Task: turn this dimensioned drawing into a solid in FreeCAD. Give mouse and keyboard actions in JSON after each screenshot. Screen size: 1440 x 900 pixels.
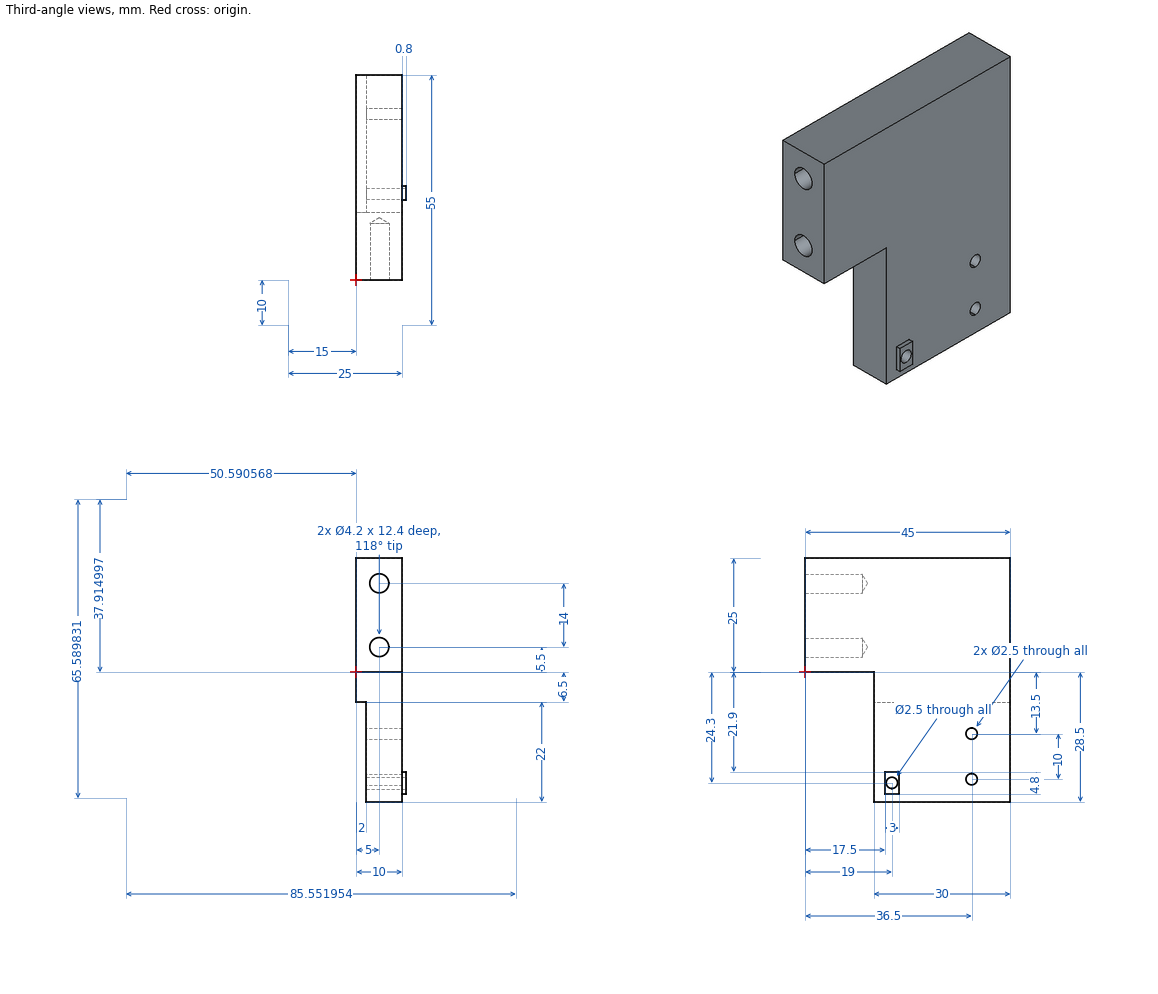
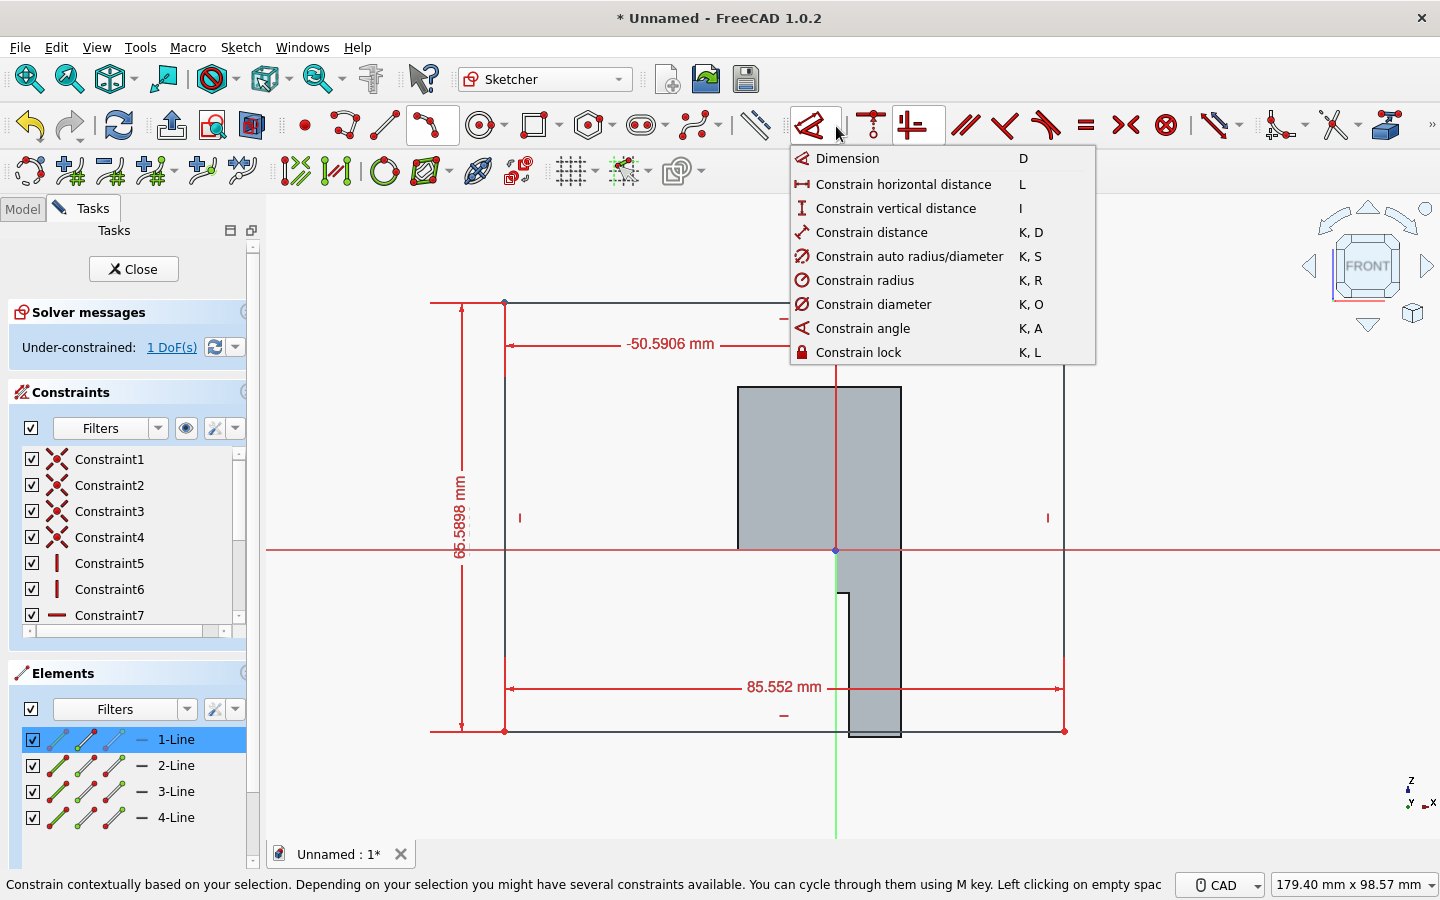
{"action": "left_click", "coordinate": [943, 208]}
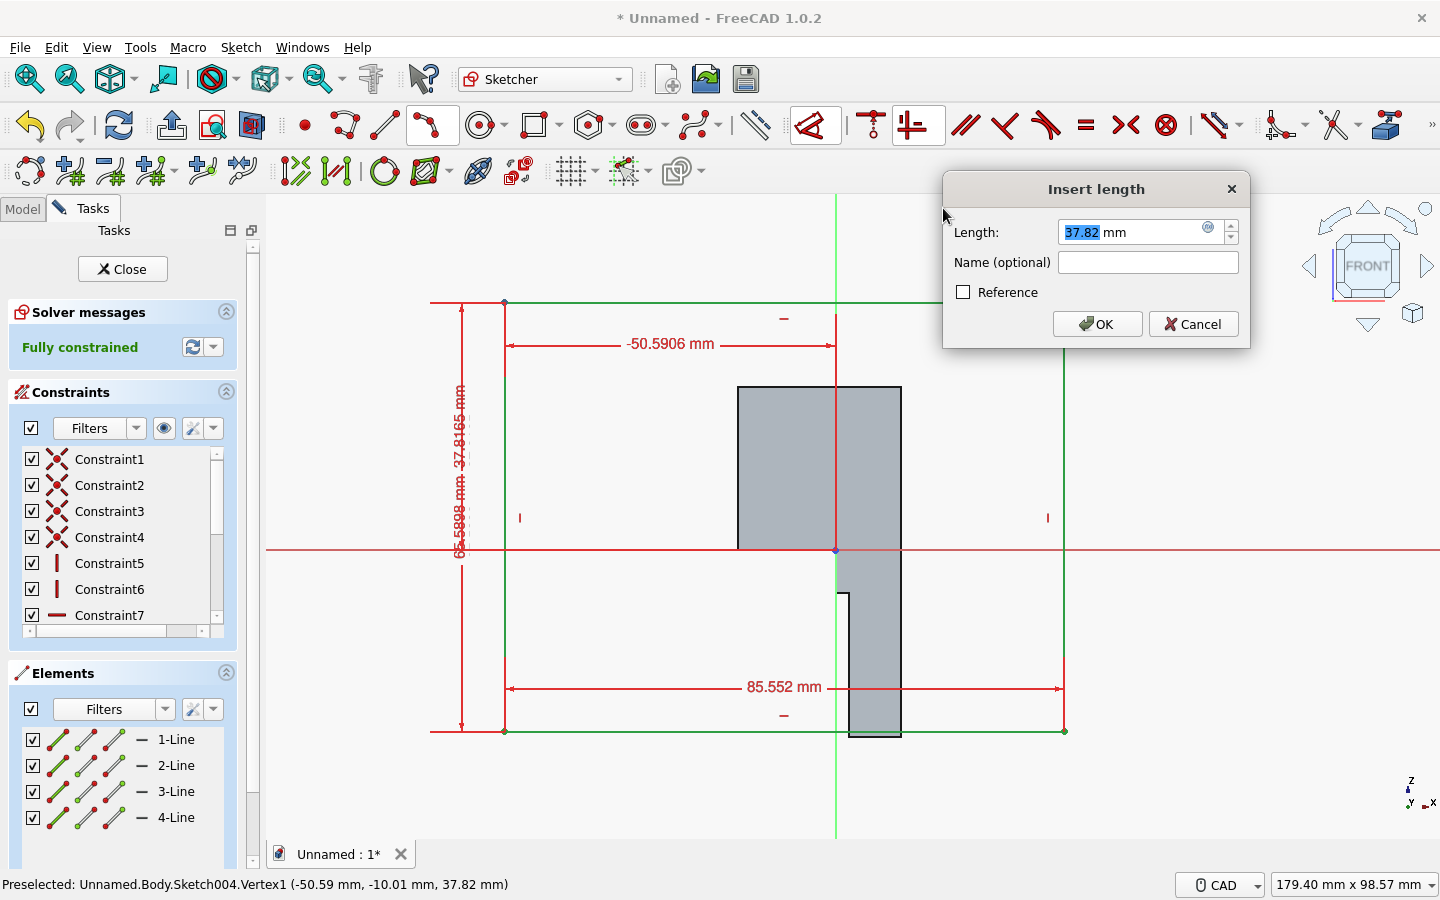
{"action": "type", "text": "37.914997"}
{"action": "key", "text": "Return"}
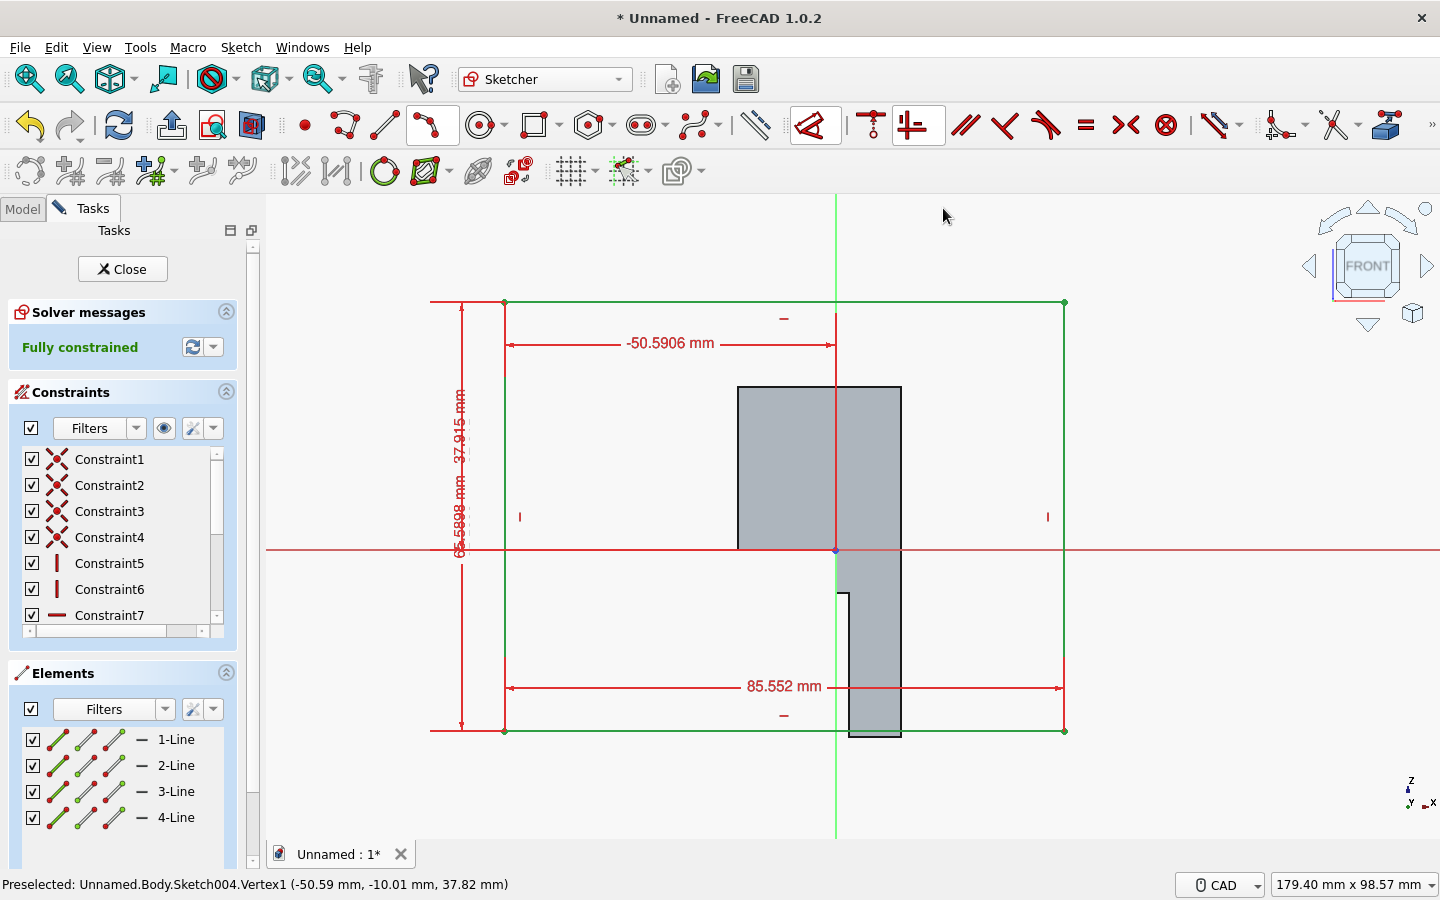
{"action": "left_click", "coordinate": [123, 269]}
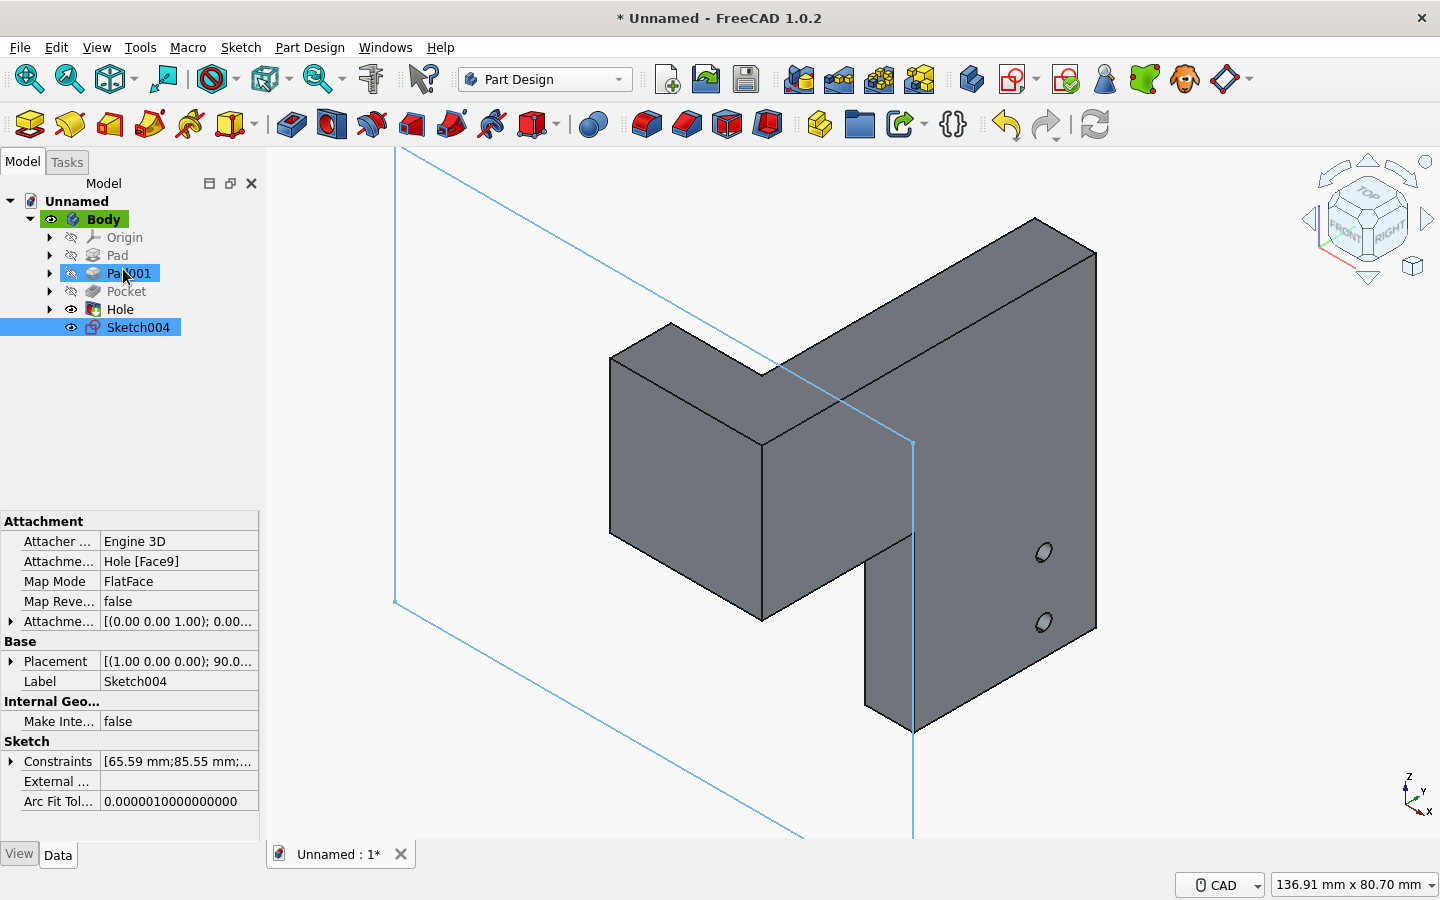
{"action": "left_click", "coordinate": [292, 124]}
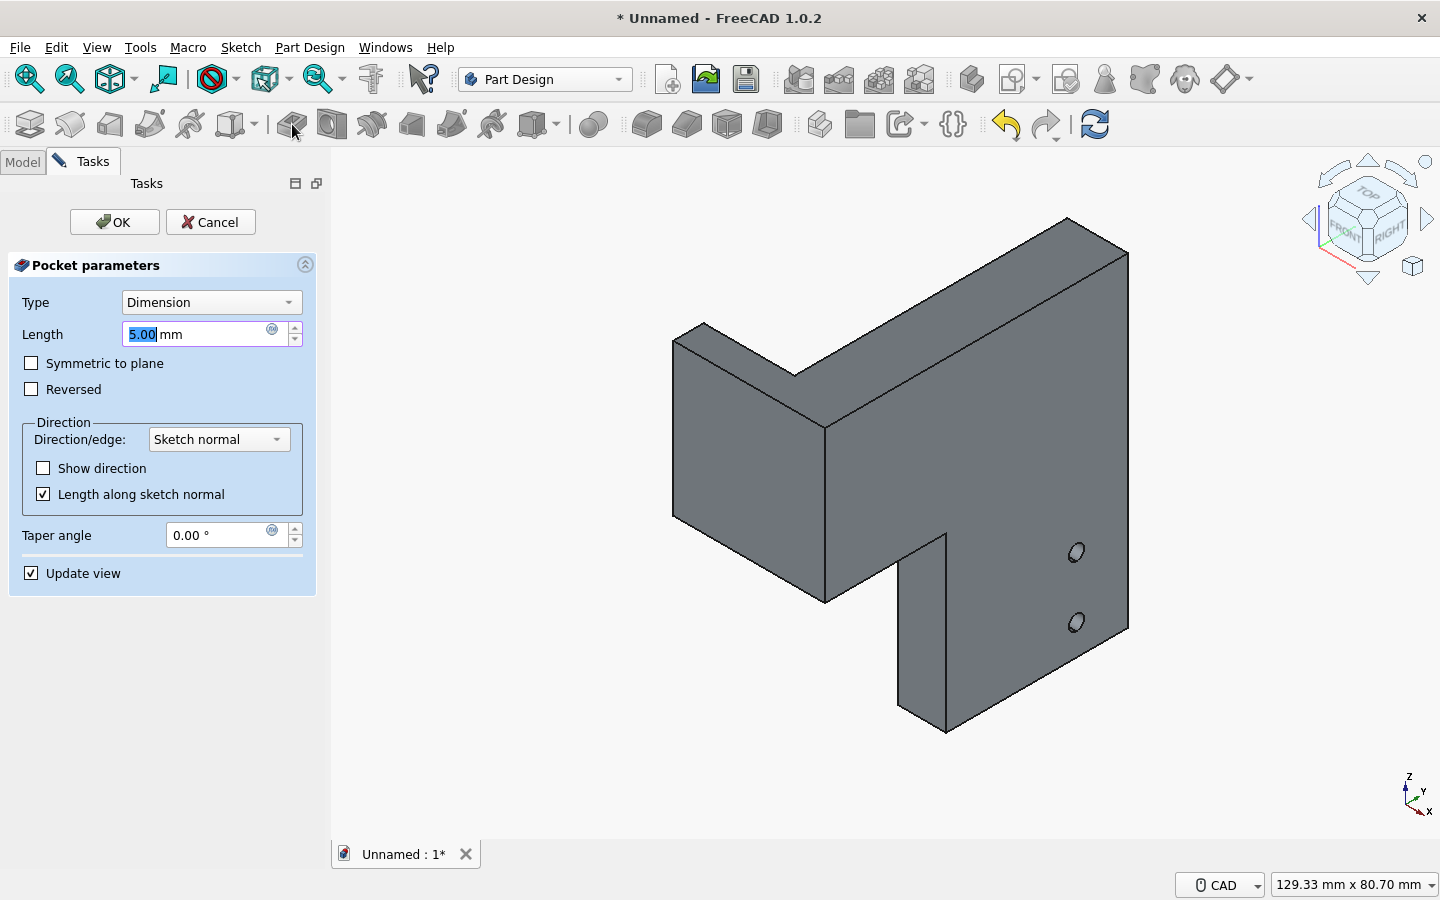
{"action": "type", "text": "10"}
{"action": "key", "text": "Tab"}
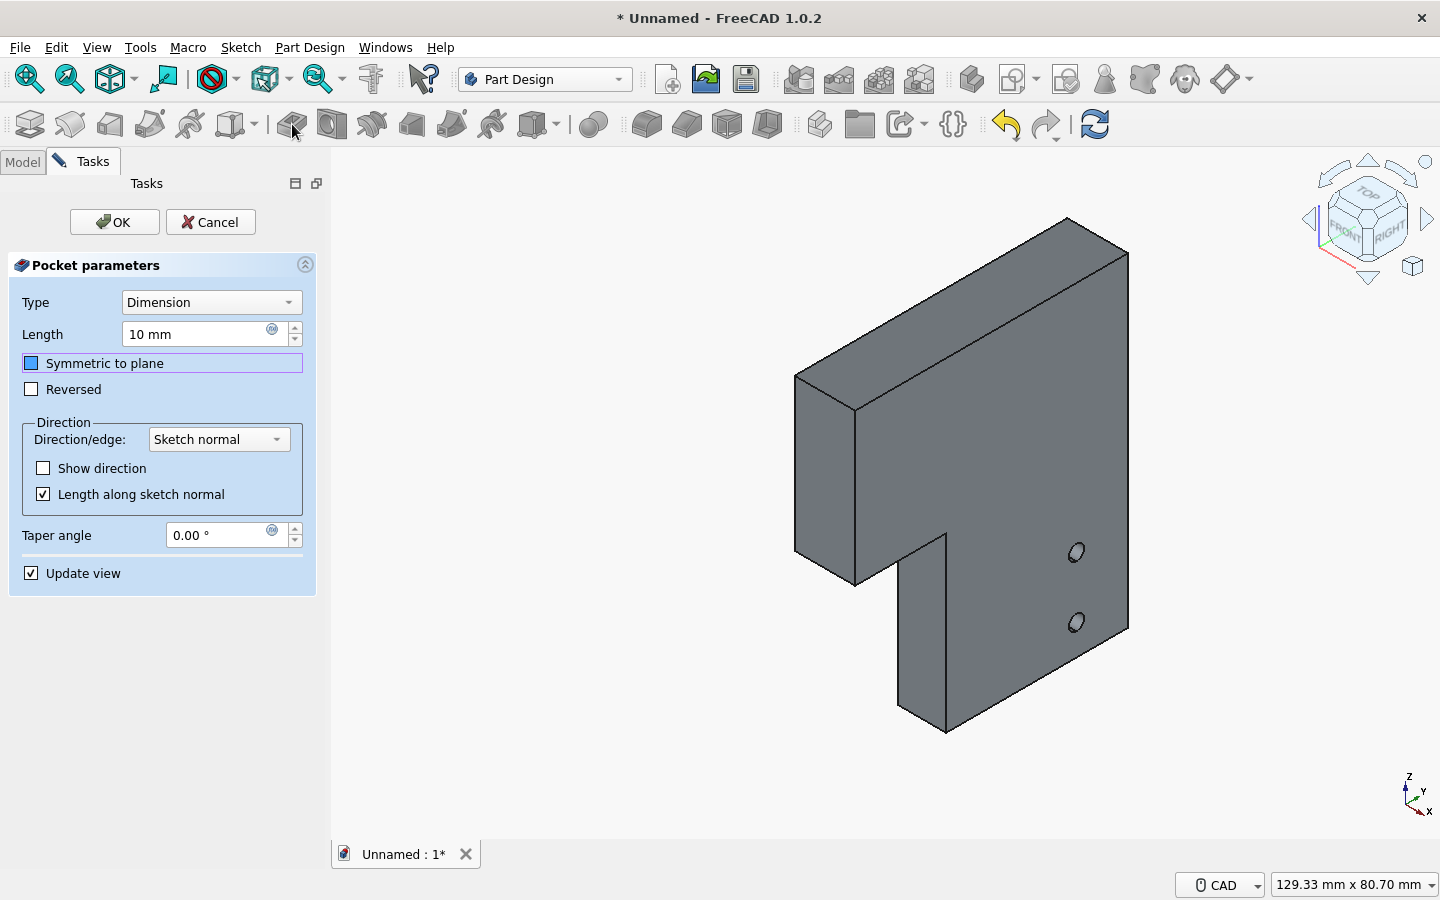
{"action": "left_click", "coordinate": [115, 222]}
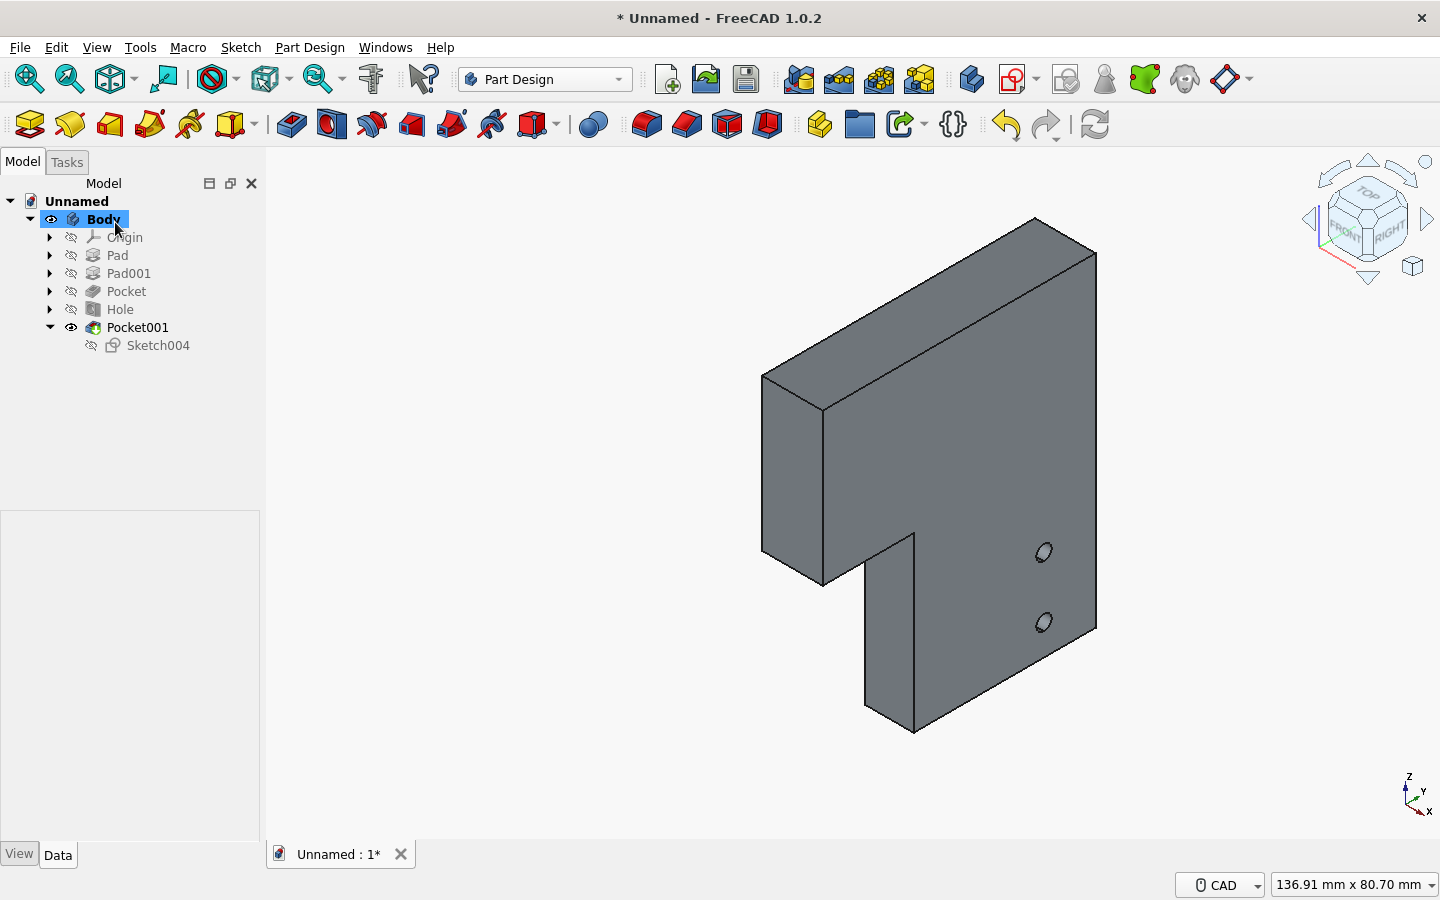
{"action": "left_click", "coordinate": [1012, 80]}